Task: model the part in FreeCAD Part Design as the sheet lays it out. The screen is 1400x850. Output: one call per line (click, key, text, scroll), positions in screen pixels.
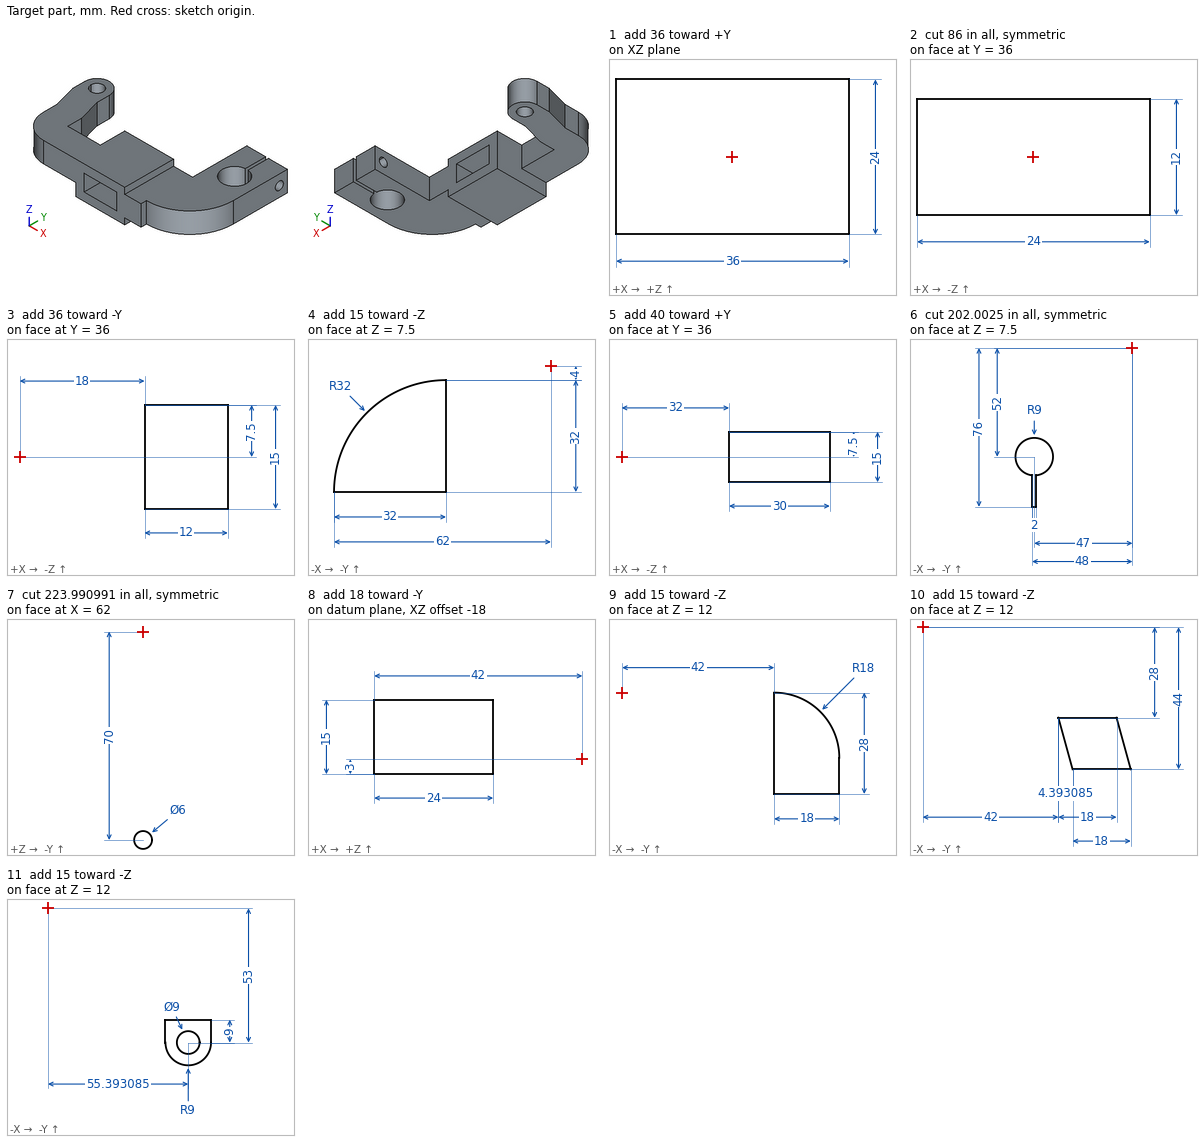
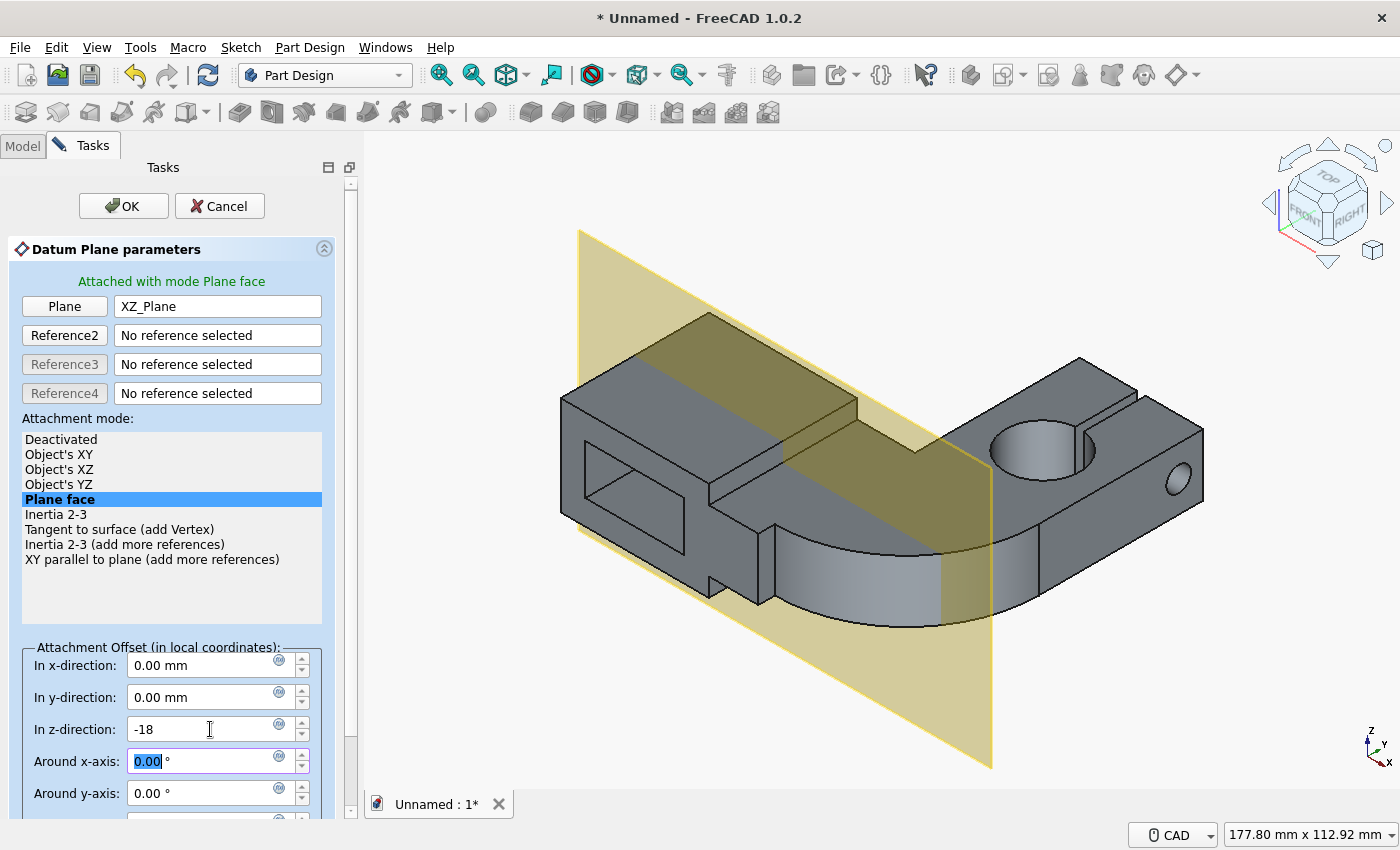
click(124, 206)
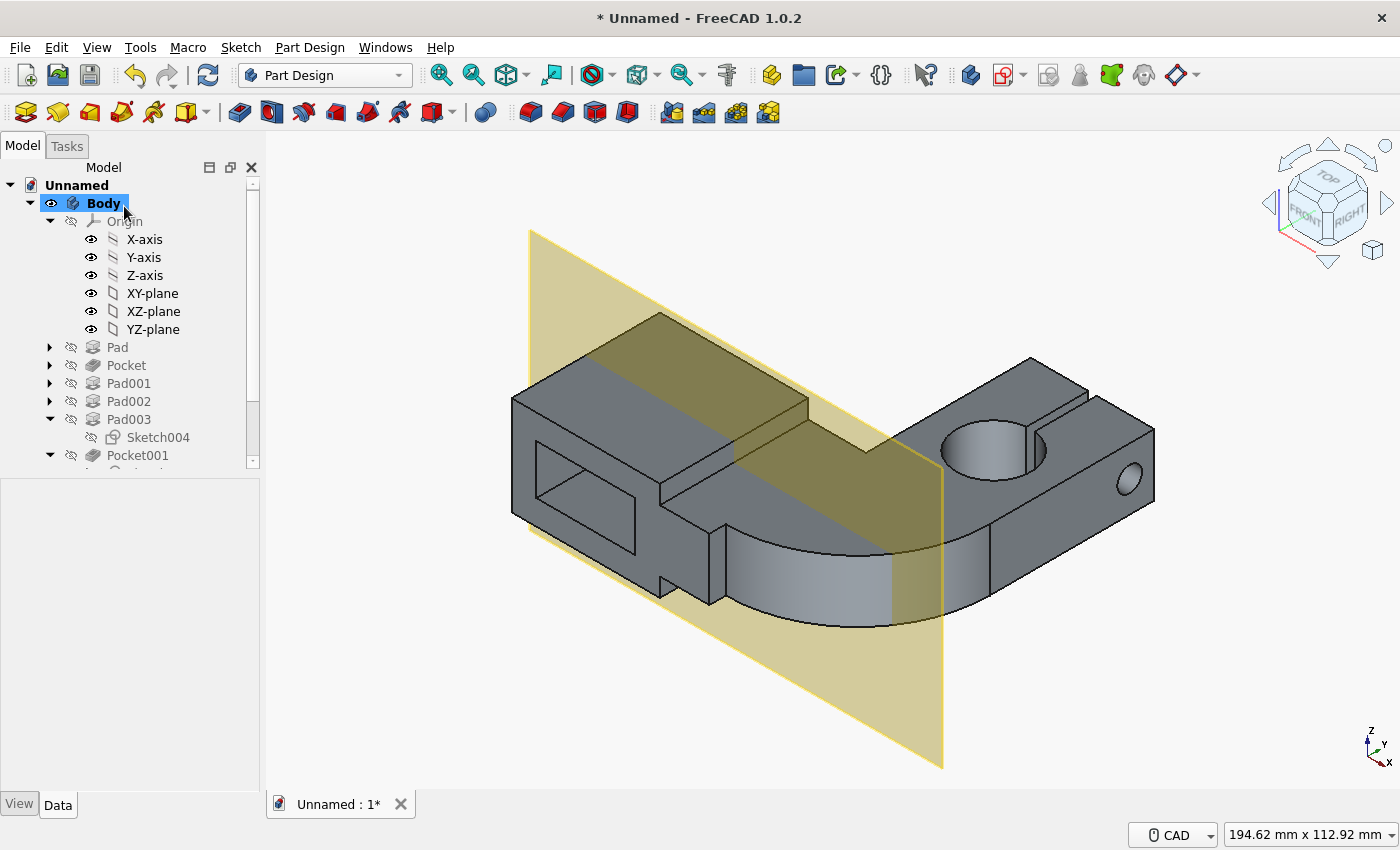
scroll(100, 325, down, 3)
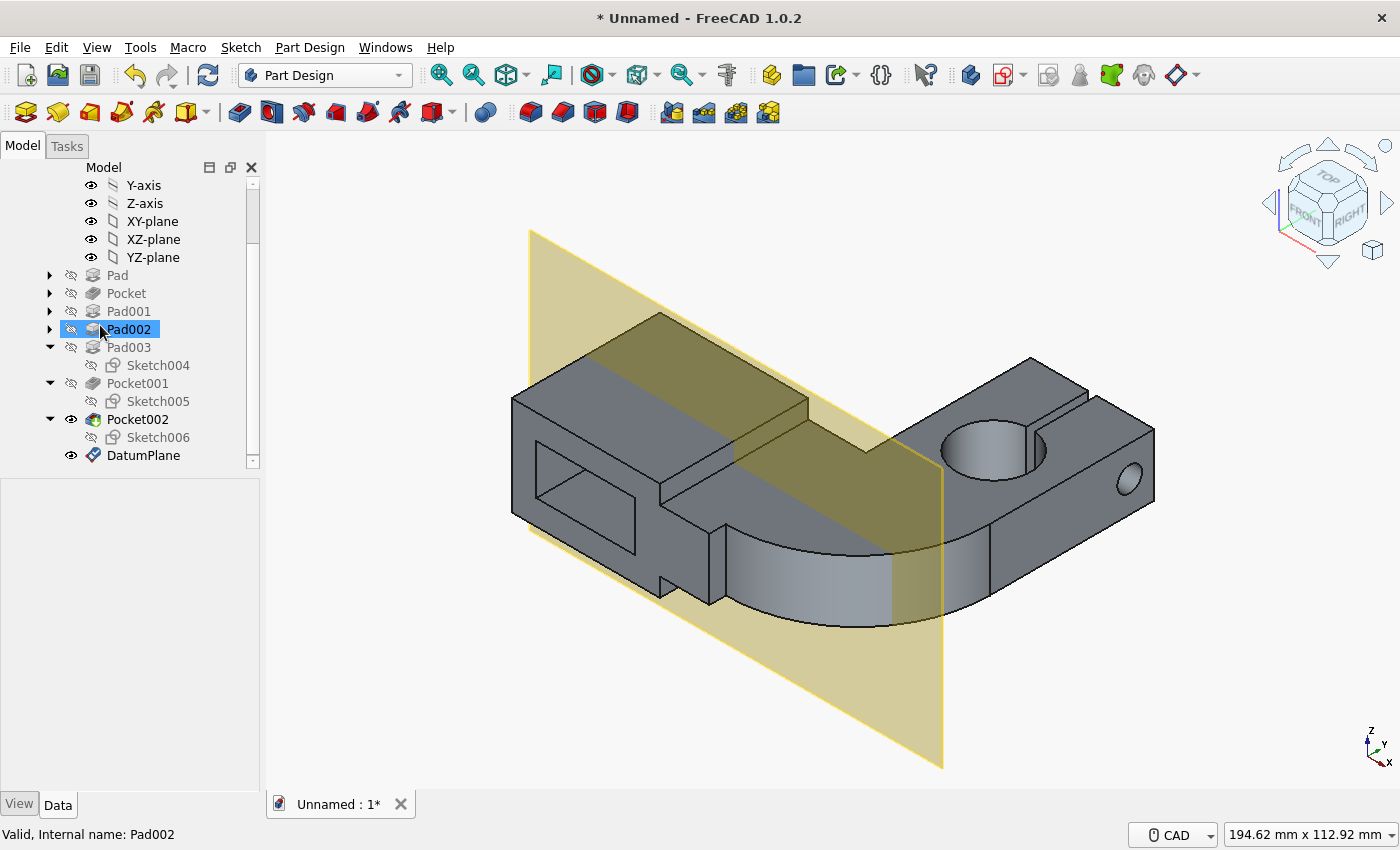
click(116, 455)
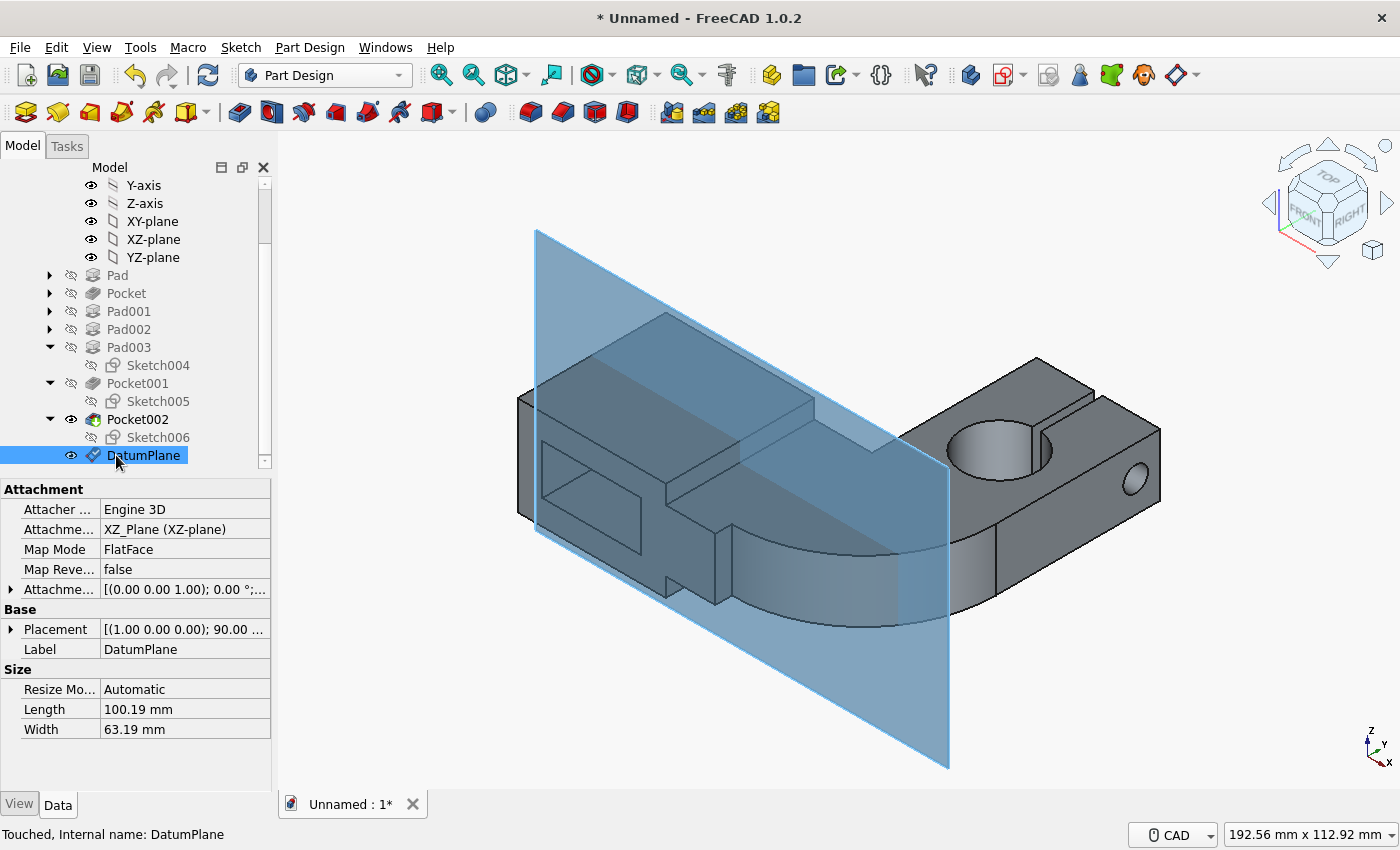
click(1004, 76)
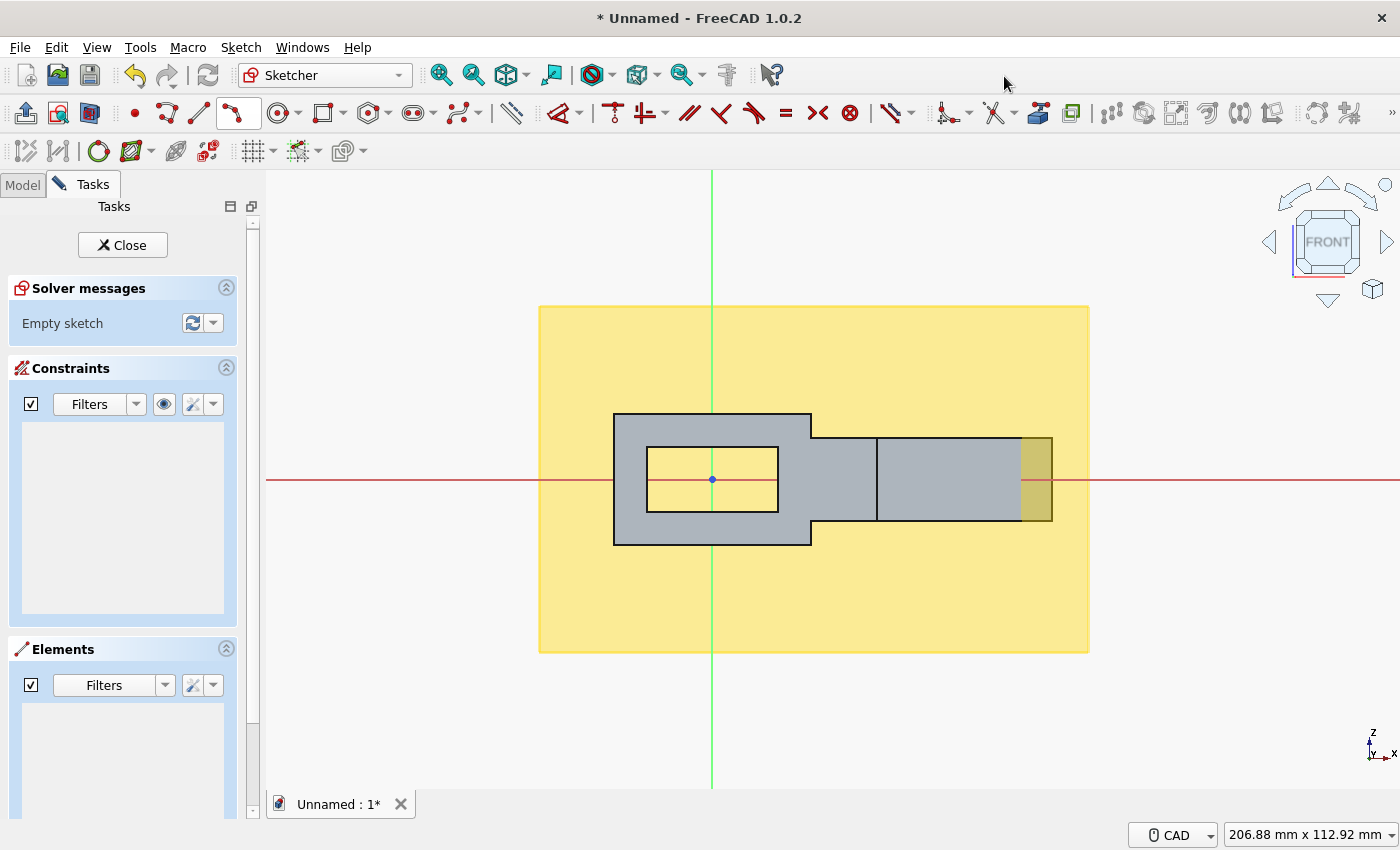
key(q)
key(s)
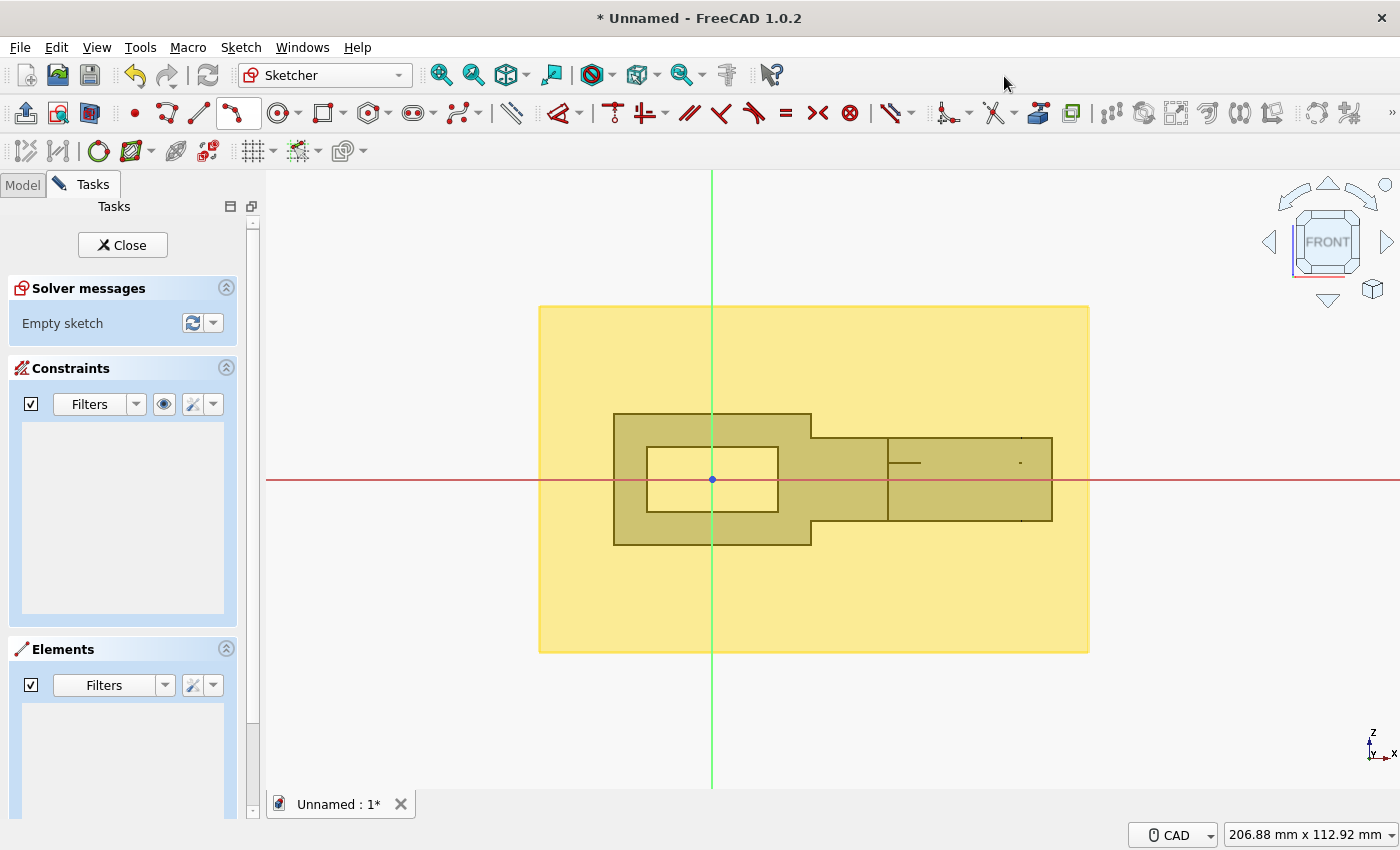
scroll(500, 440, up, 5)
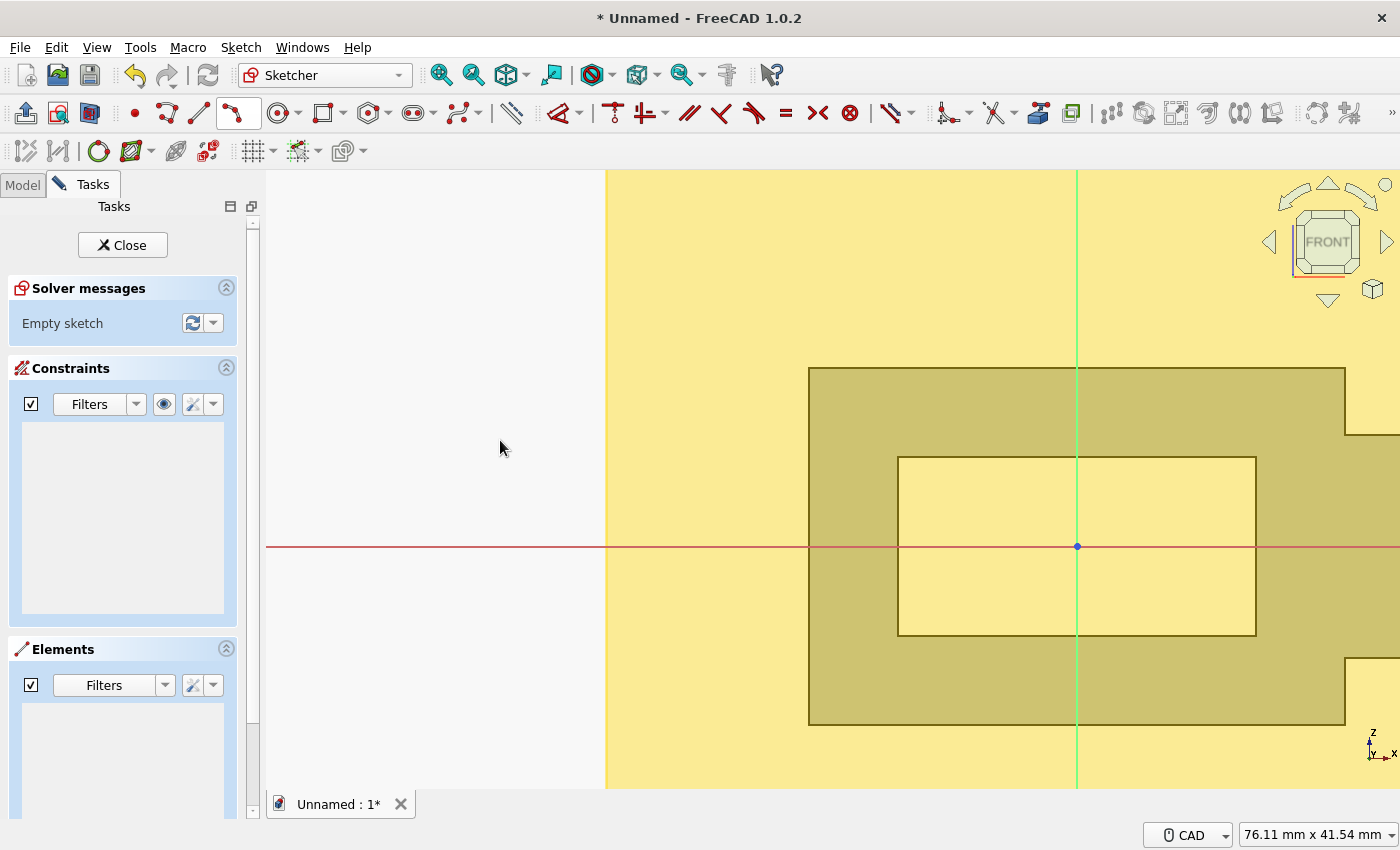
key(g)
key(r)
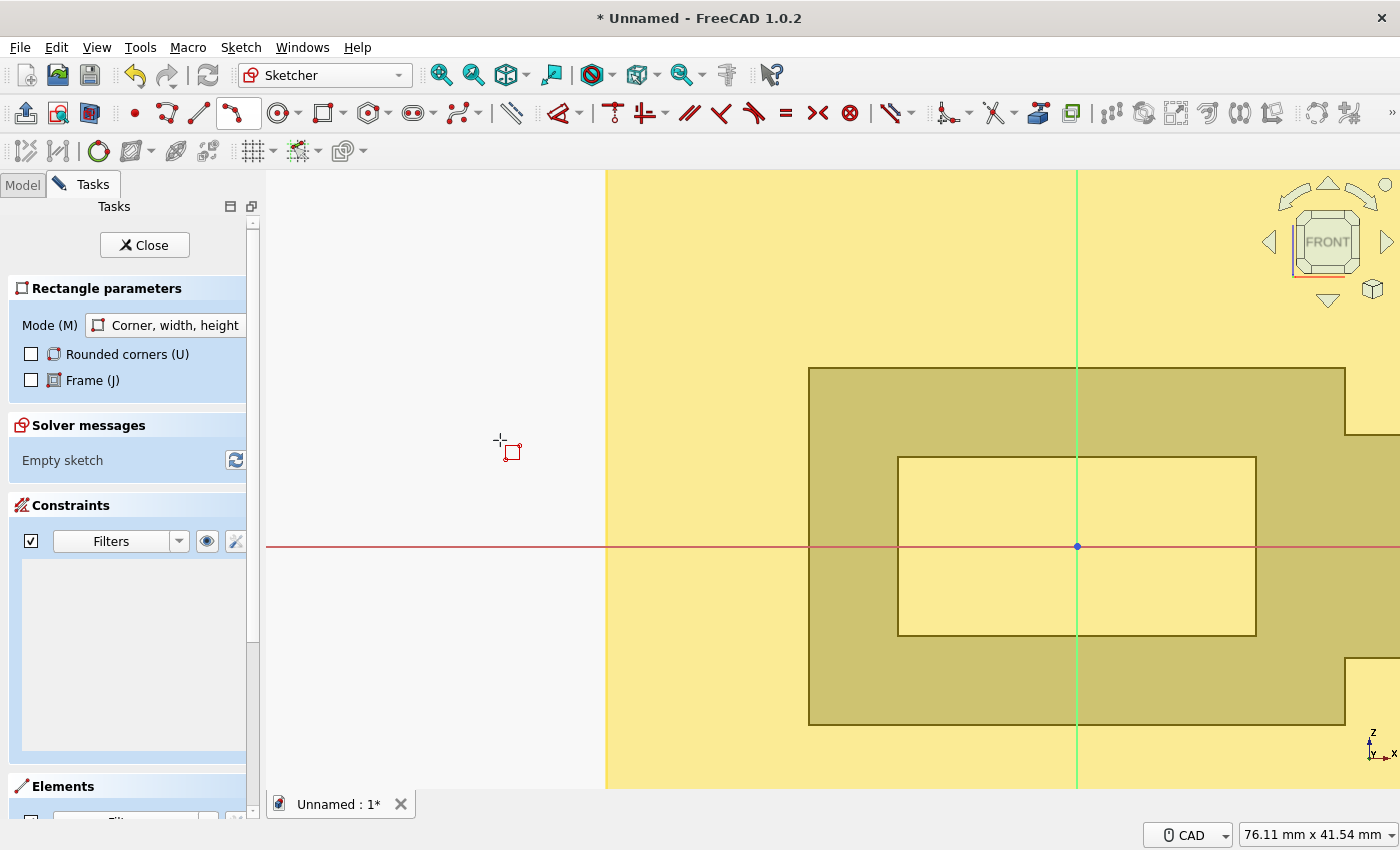
click(451, 368)
click(809, 591)
key(Escape)